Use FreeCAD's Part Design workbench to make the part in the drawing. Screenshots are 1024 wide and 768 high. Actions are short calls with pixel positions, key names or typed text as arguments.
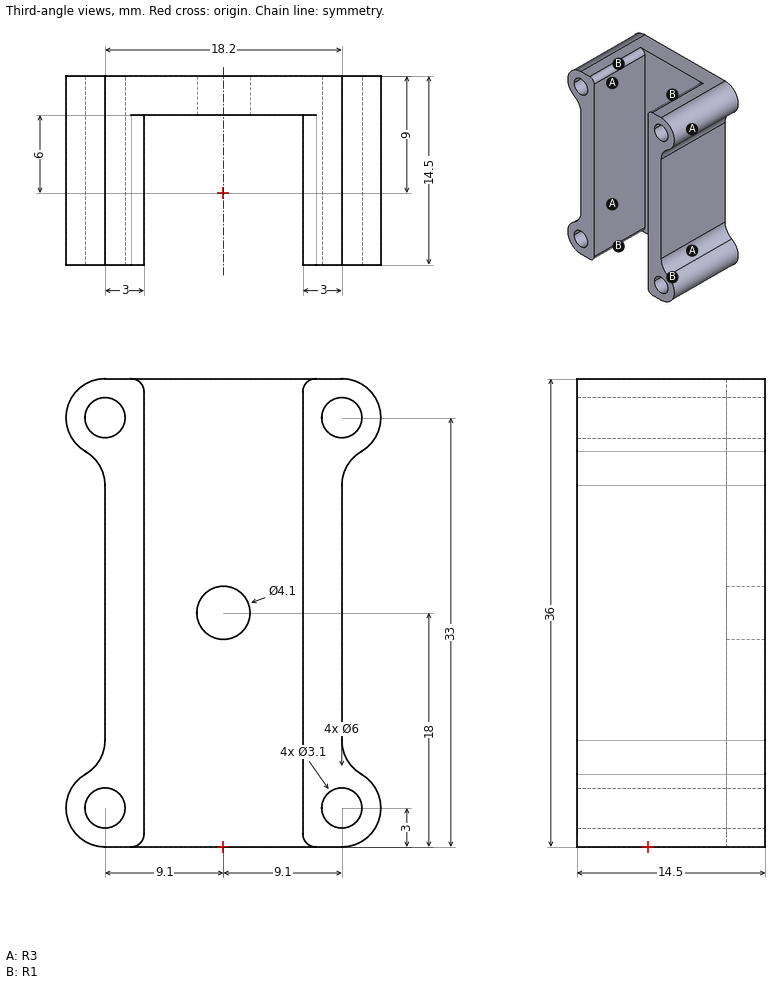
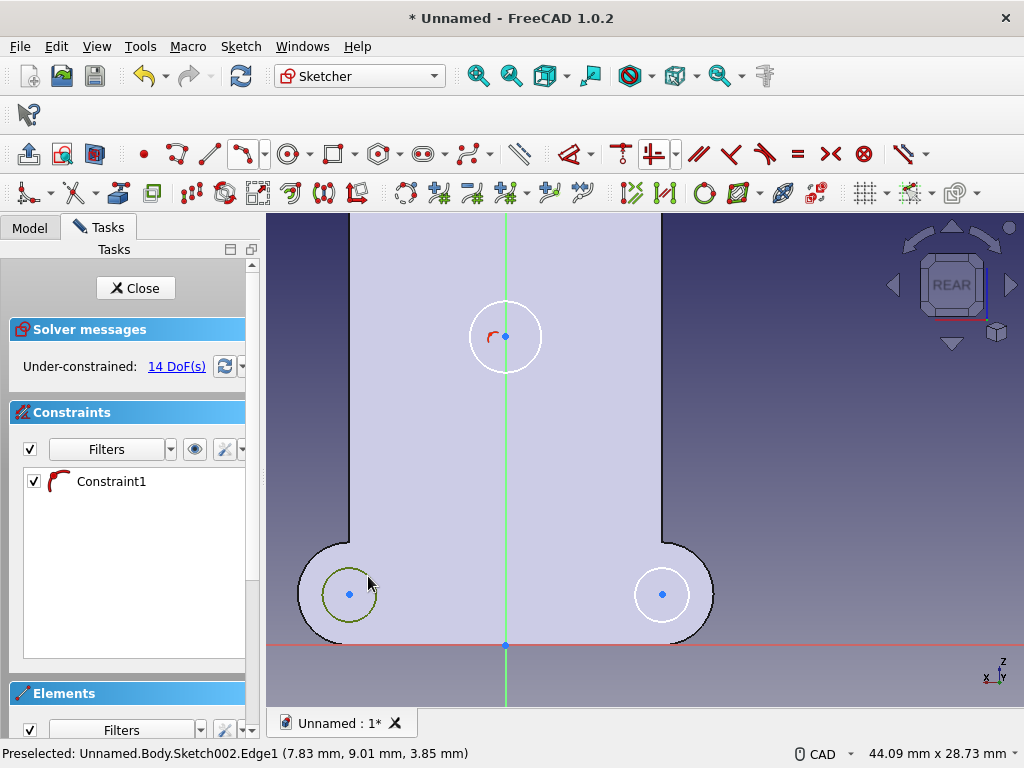
scroll(663, 596, down, 3)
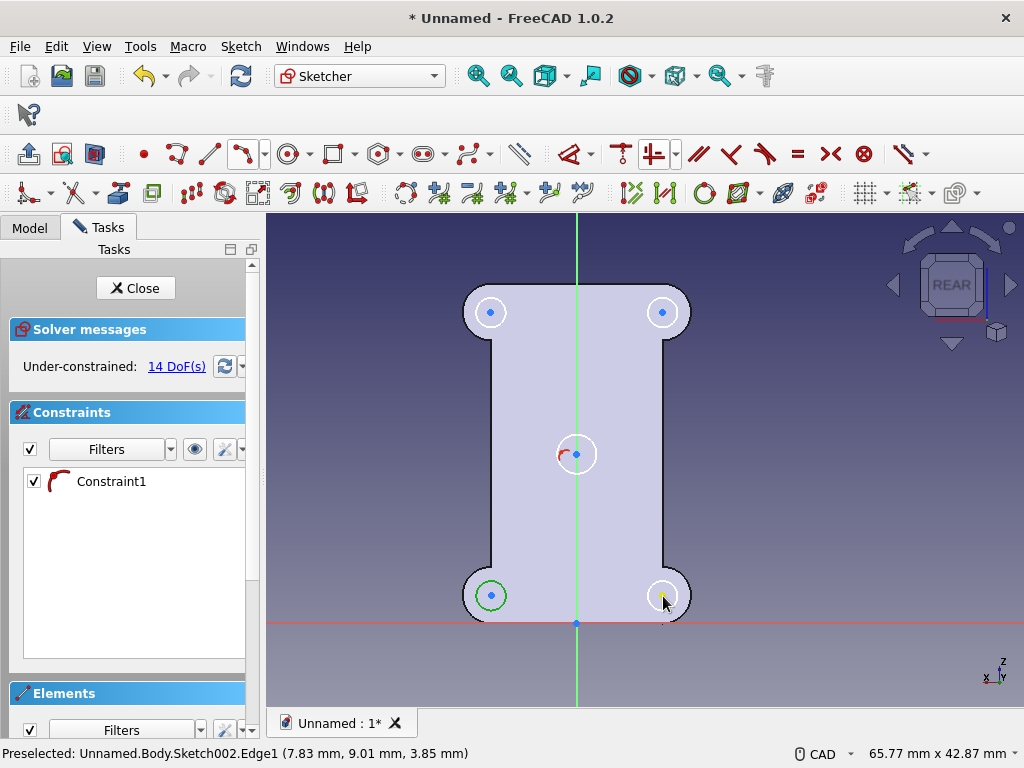
click(673, 302)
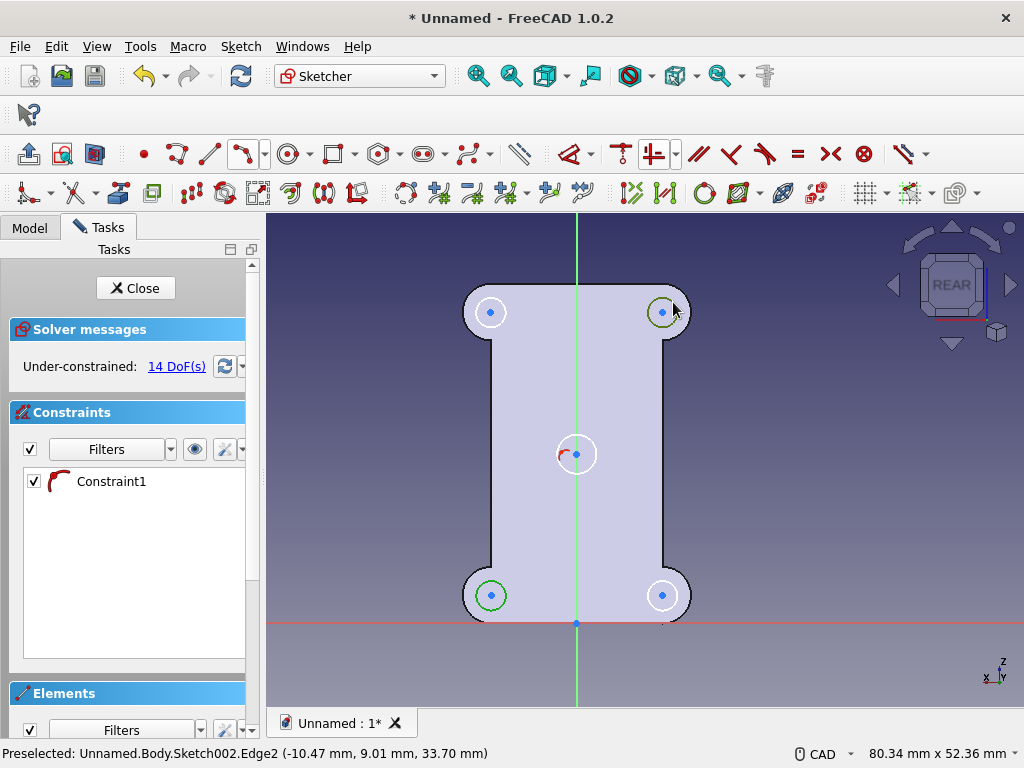
click(501, 302)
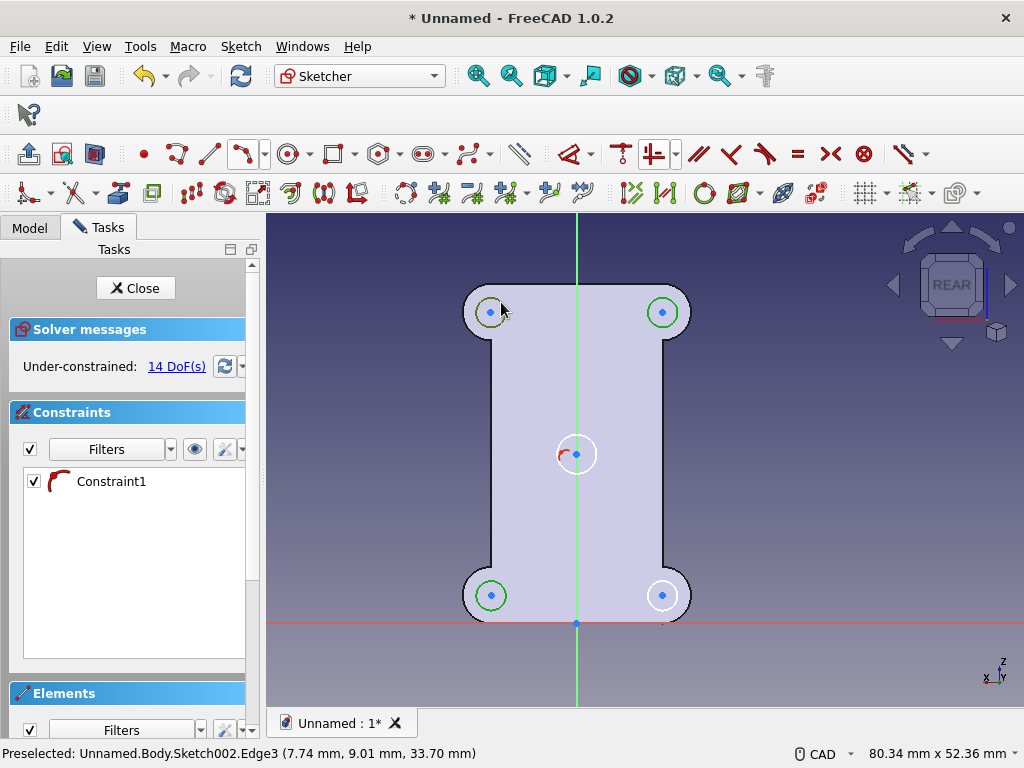
click(673, 585)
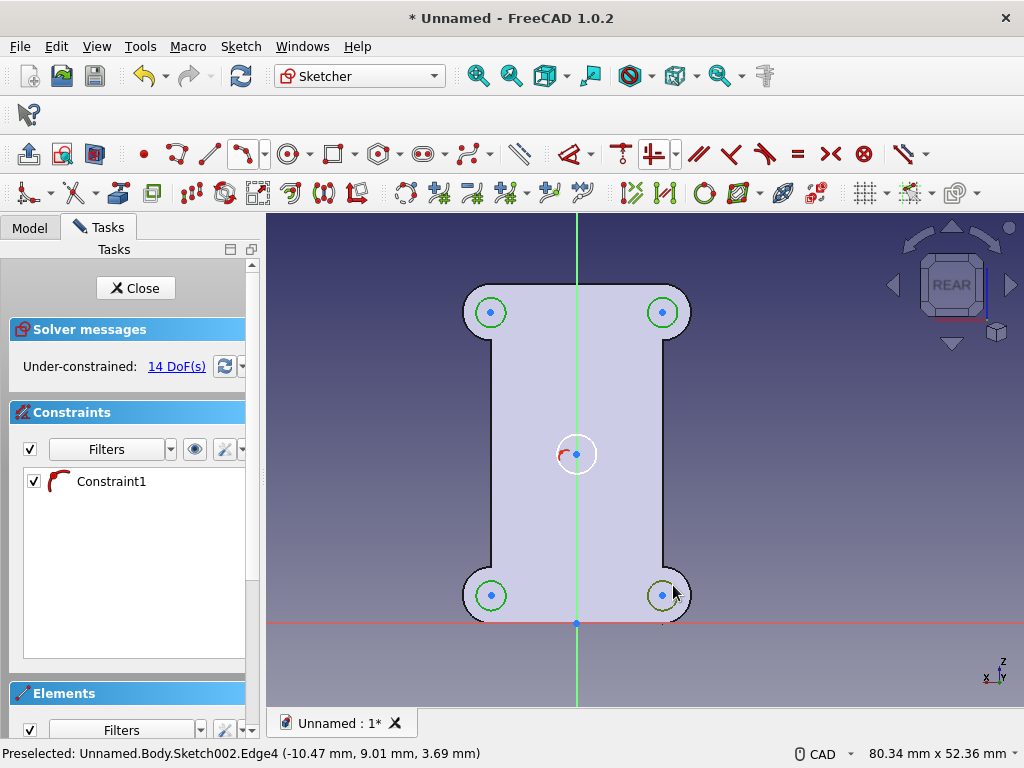
click(798, 154)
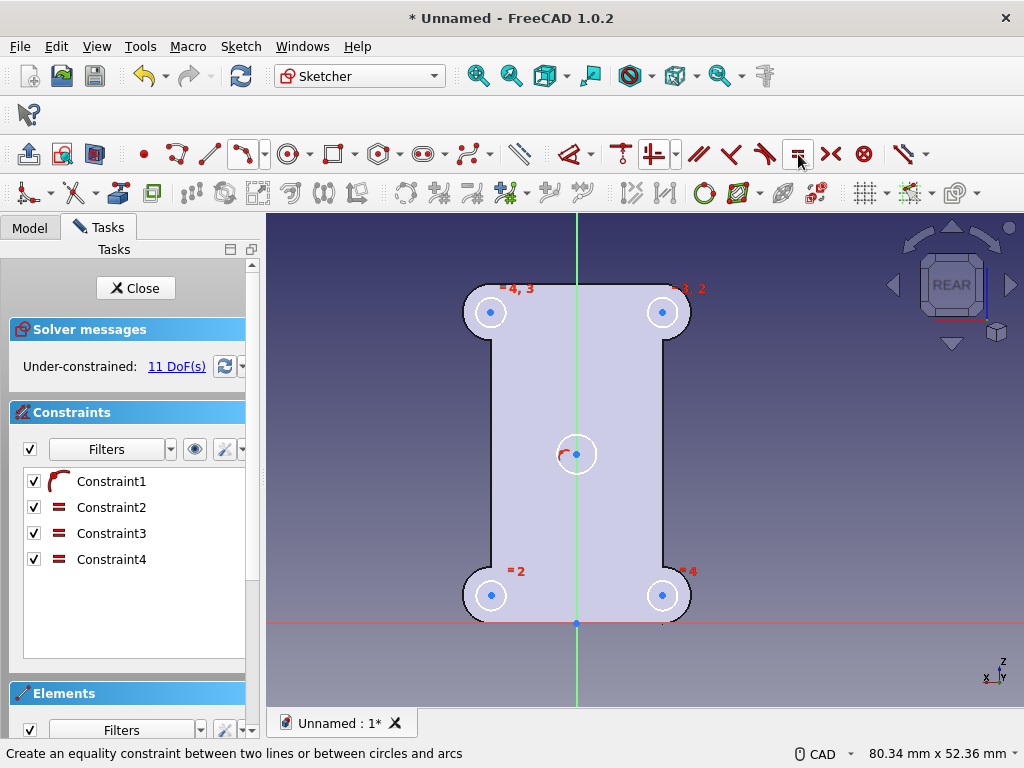
click(491, 596)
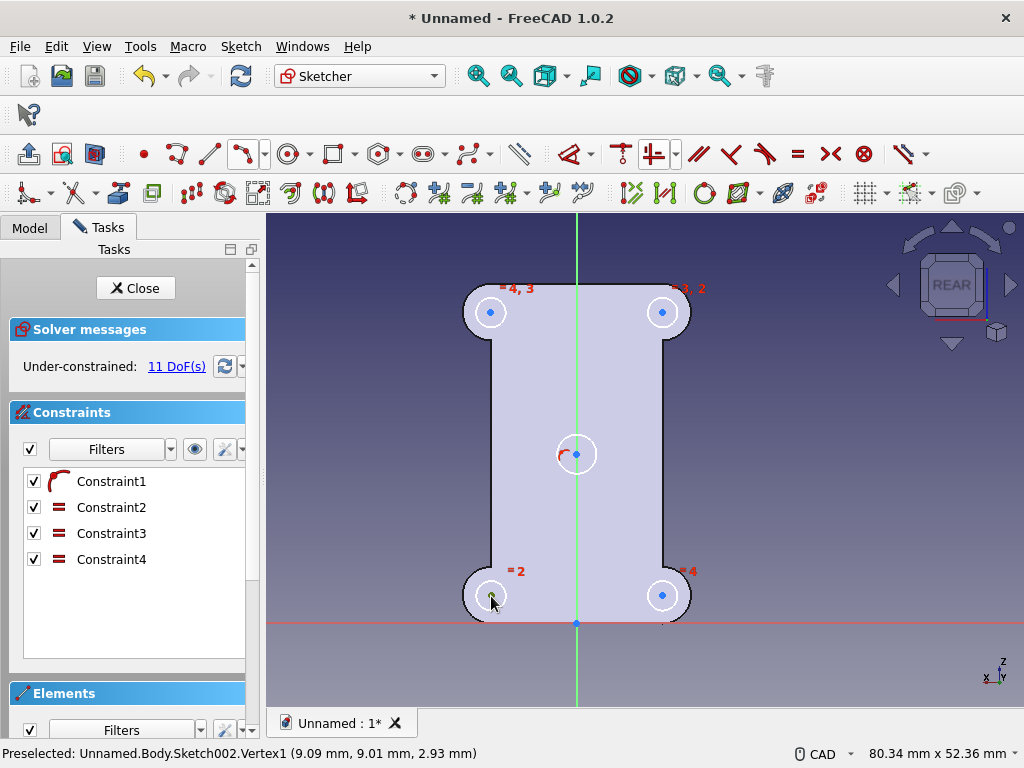
click(491, 313)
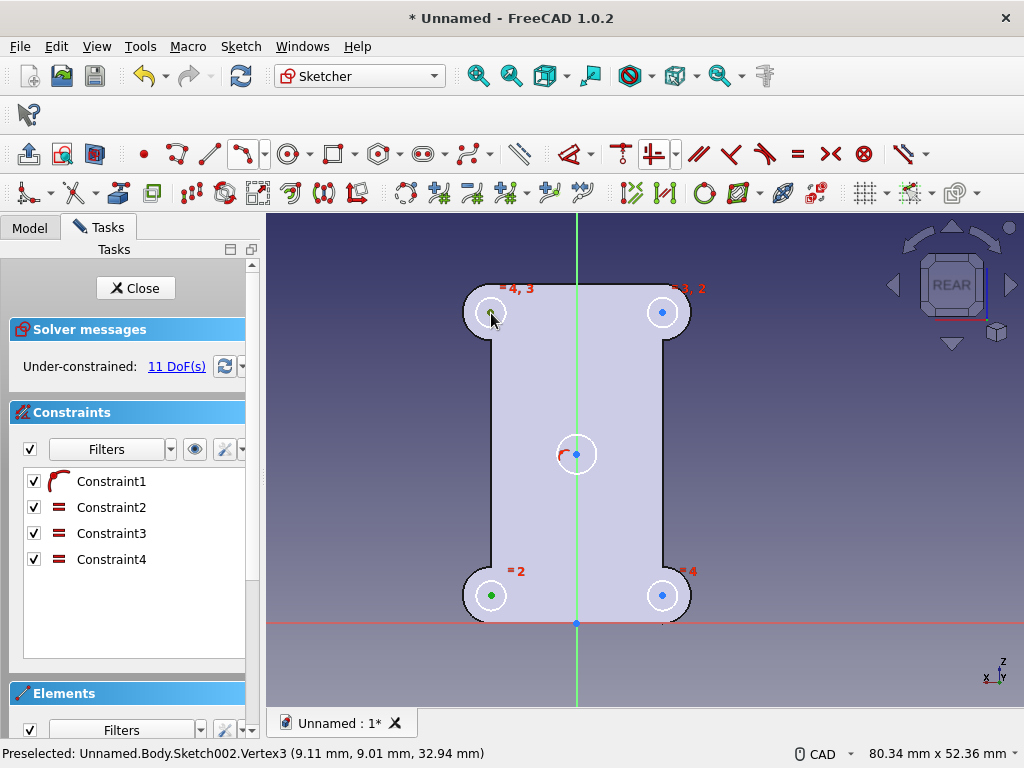
key(v)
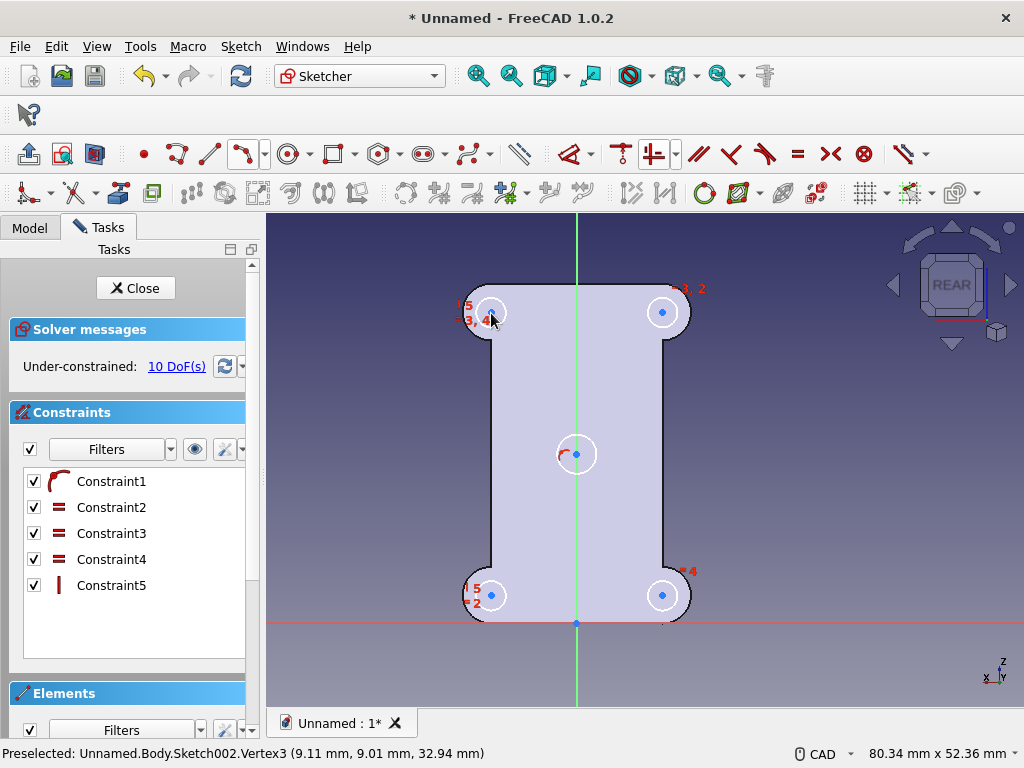
click(663, 313)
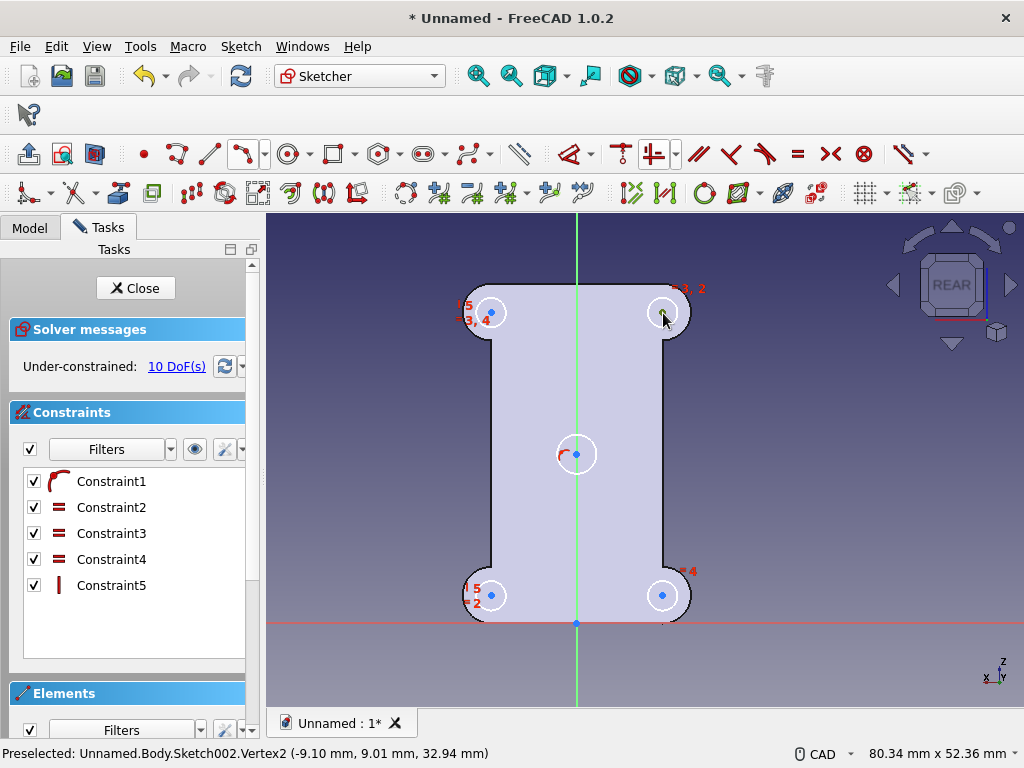
click(491, 313)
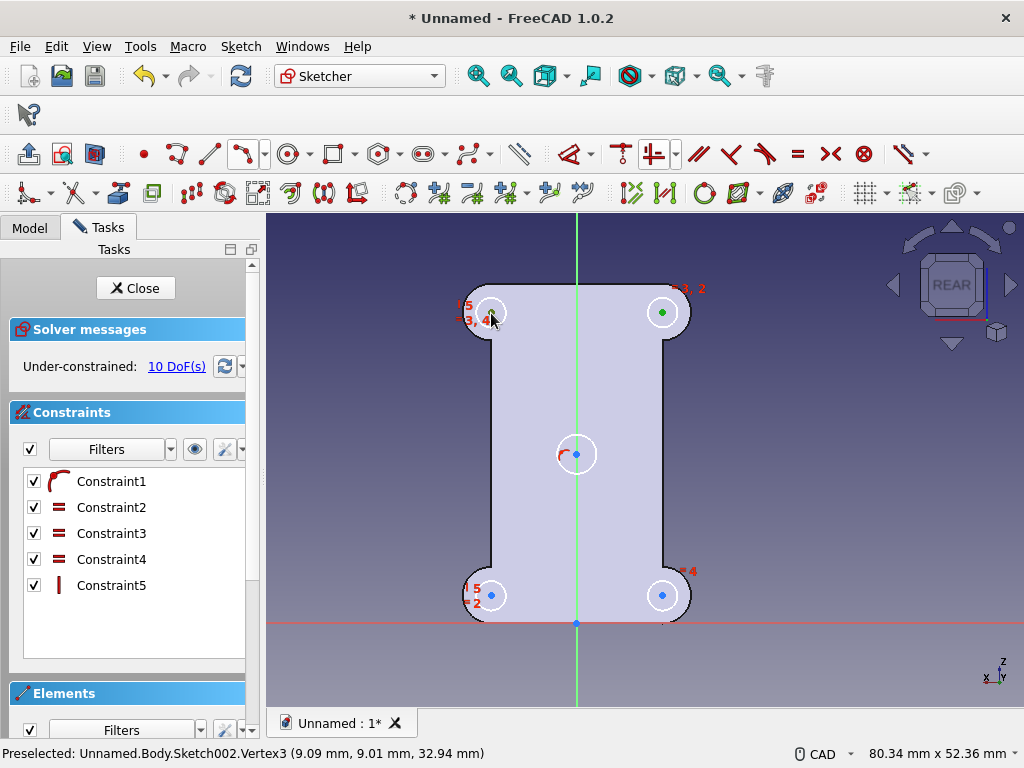
click(676, 154)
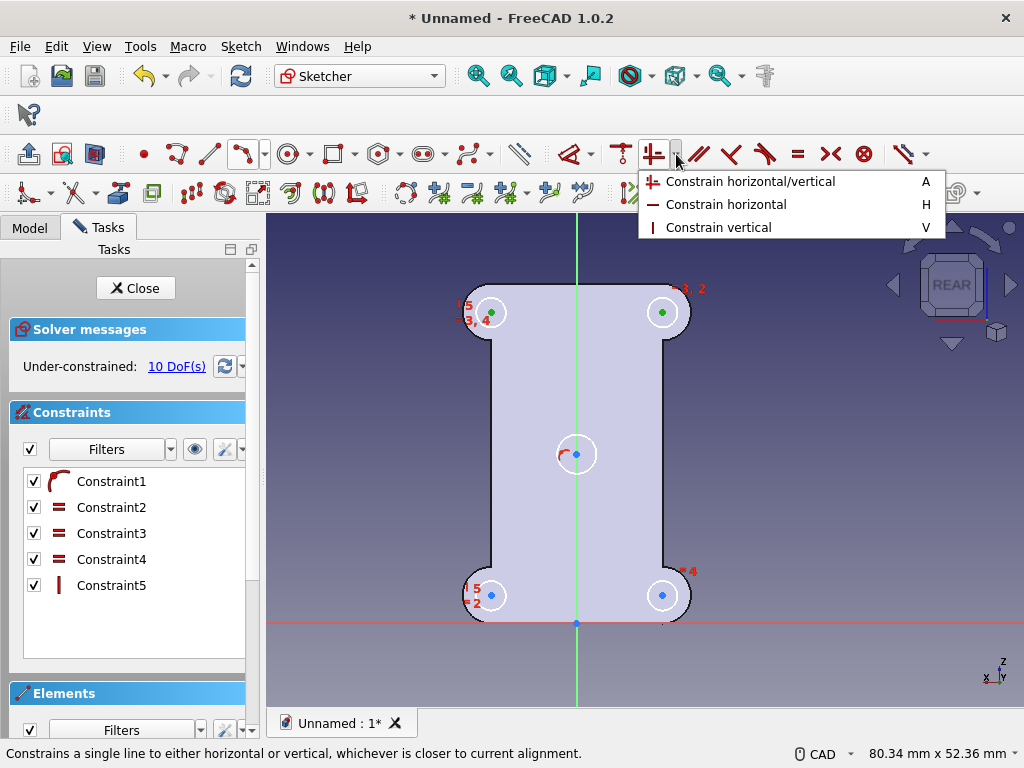
click(792, 204)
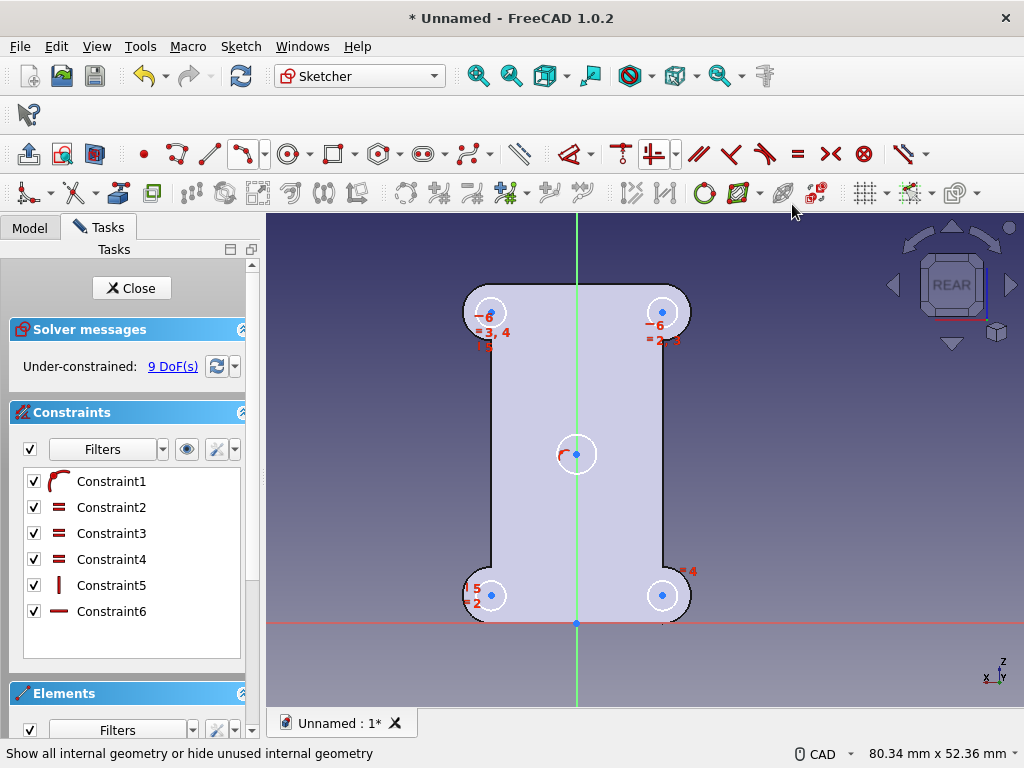
click(663, 313)